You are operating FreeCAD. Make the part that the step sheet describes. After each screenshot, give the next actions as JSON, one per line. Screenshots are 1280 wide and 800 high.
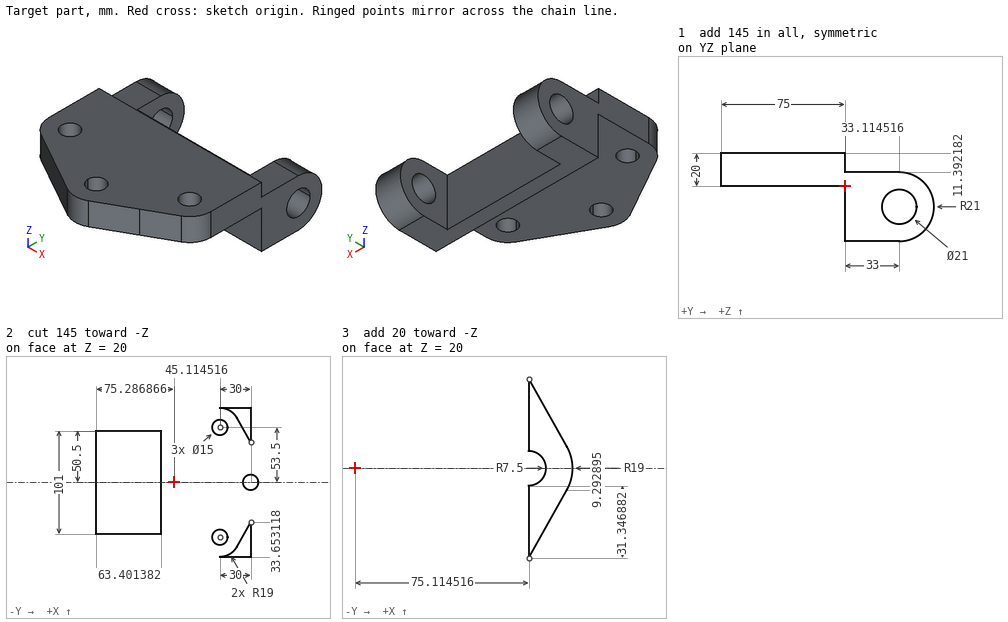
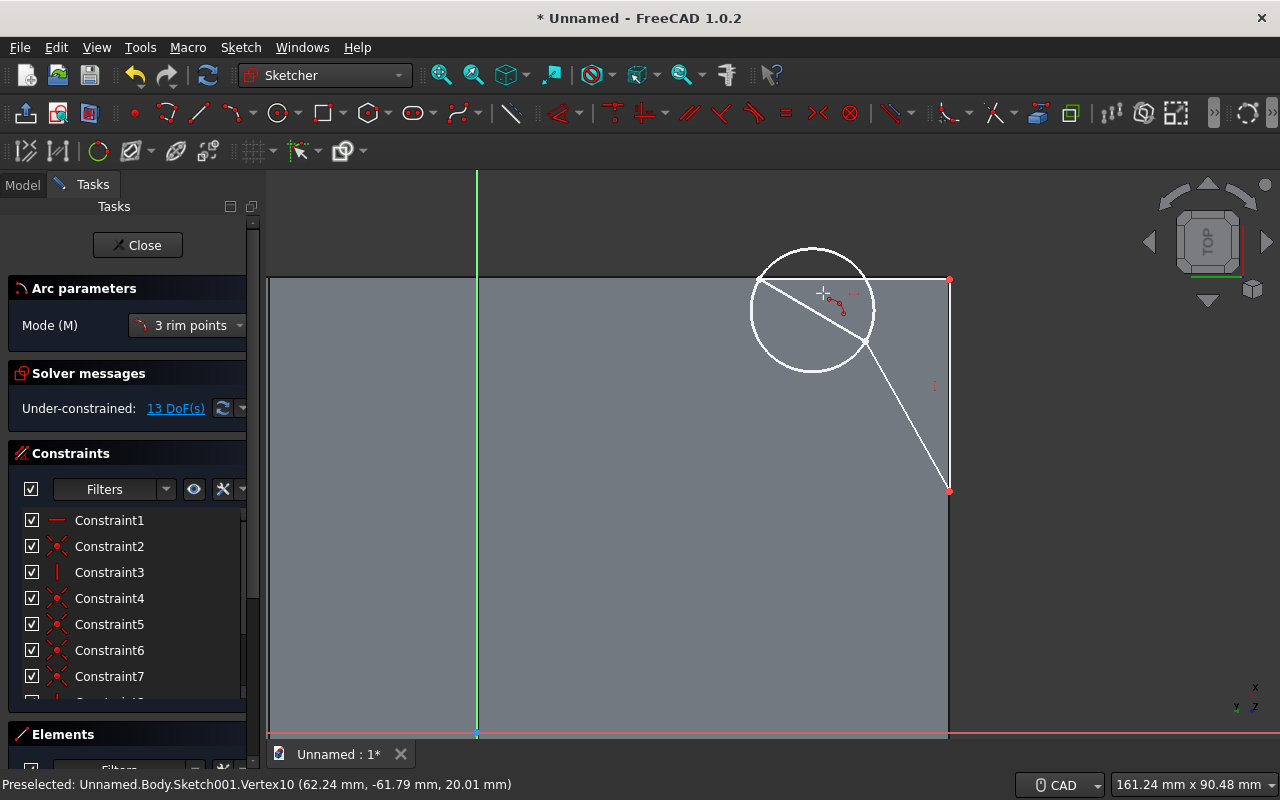
{"action": "left_click", "coordinate": [821, 293]}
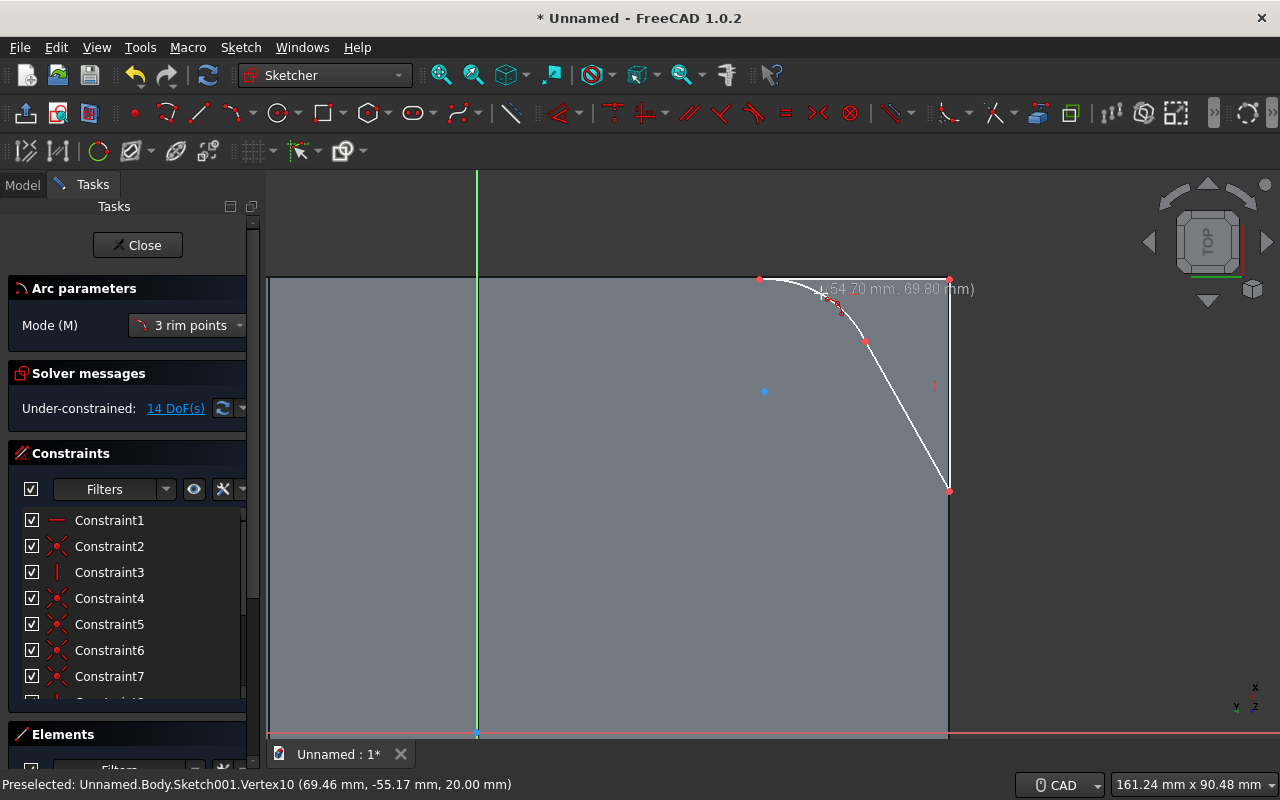
{"action": "left_click", "coordinate": [324, 114]}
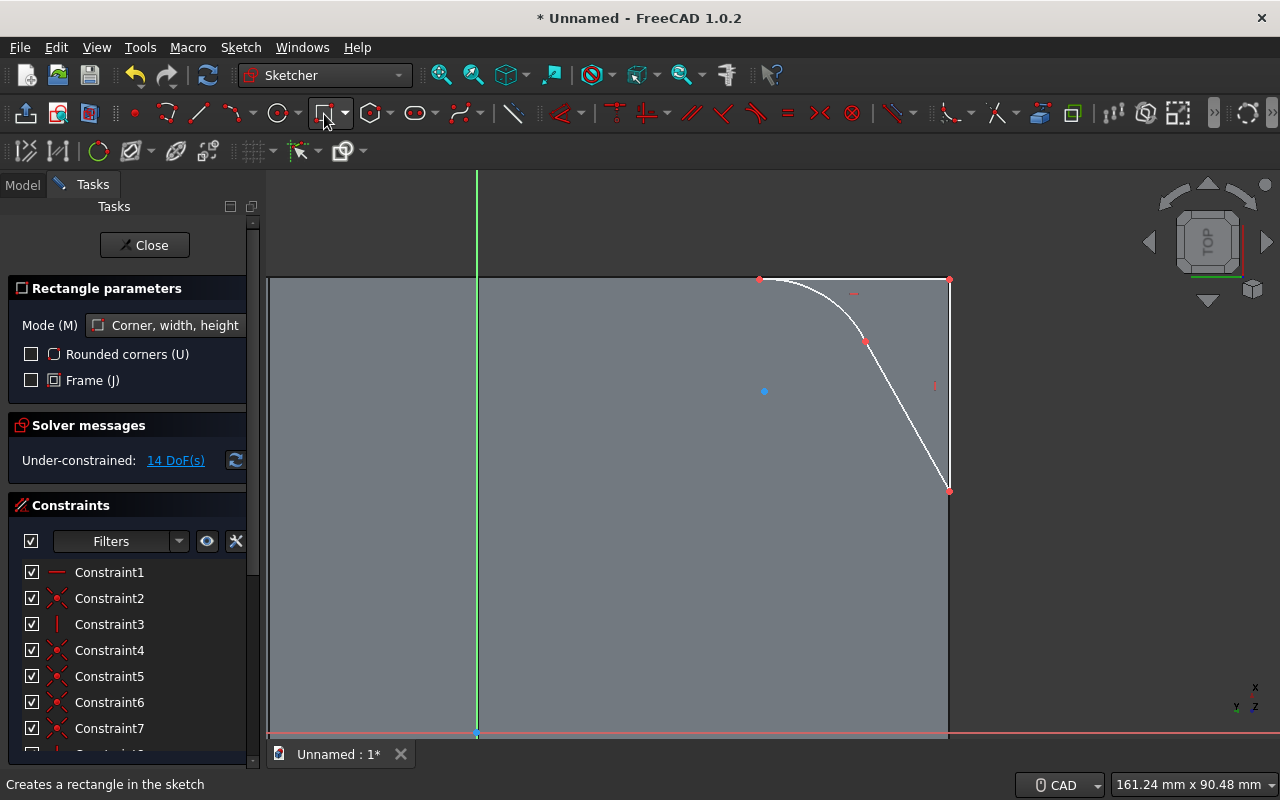
{"action": "scroll", "coordinate": [824, 292], "scroll_direction": "down", "scroll_amount": 5}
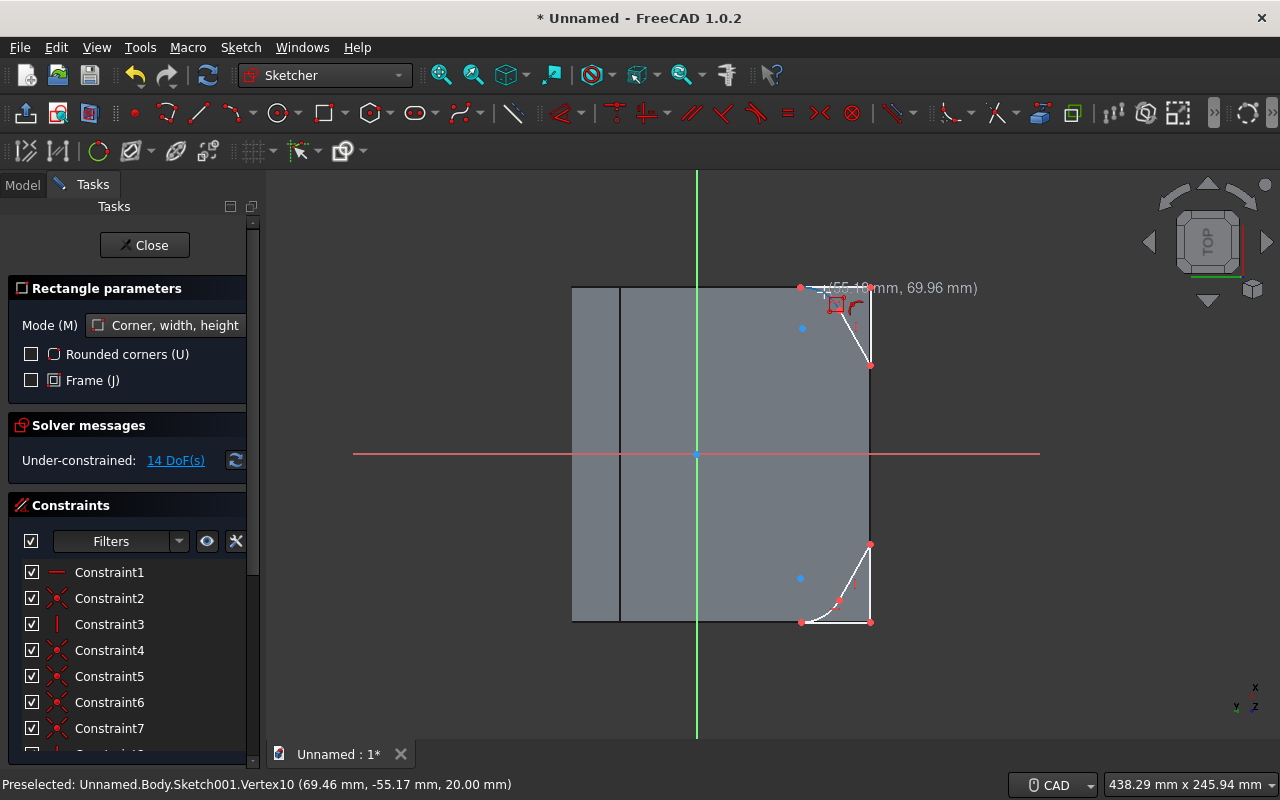
{"action": "left_click", "coordinate": [523, 338]}
{"action": "mouse_move", "coordinate": [669, 571]}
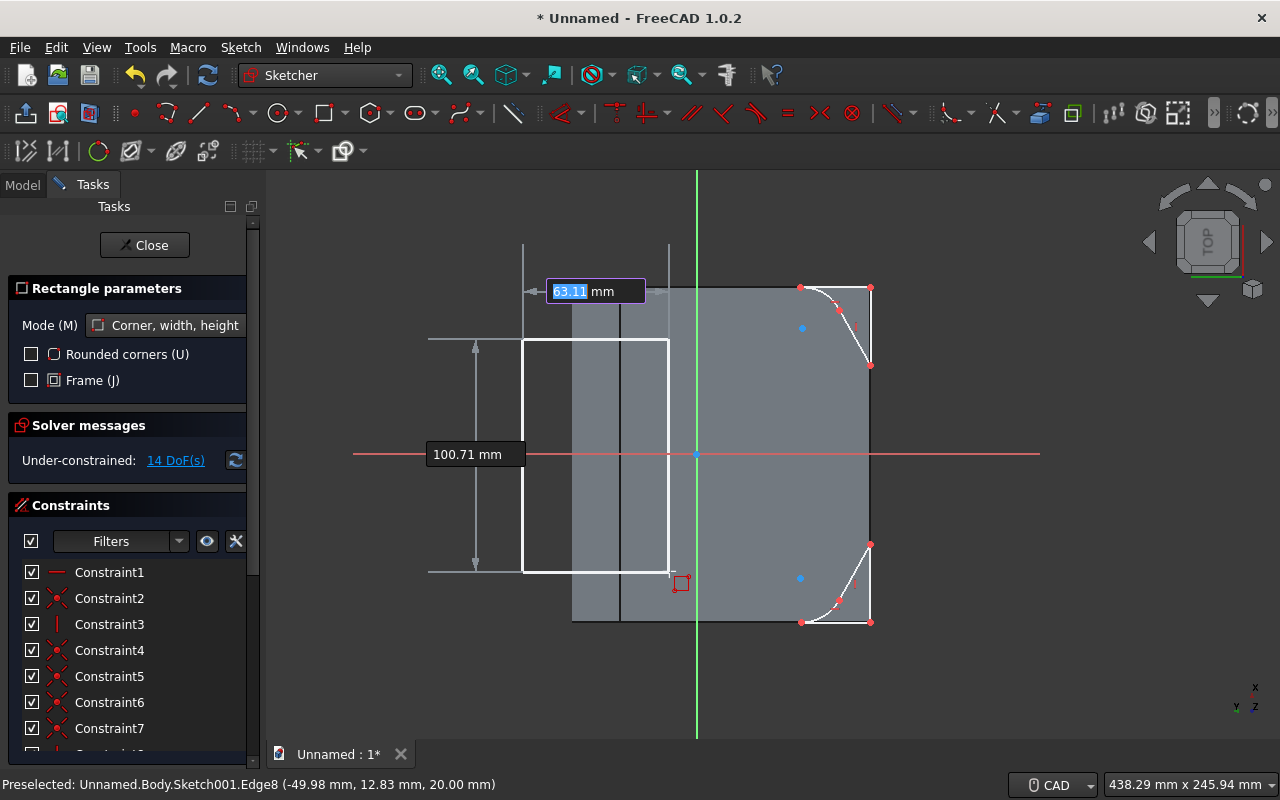
{"action": "type", "text": "63.401382"}
{"action": "key", "text": "Tab"}
{"action": "type", "text": "101"}
{"action": "key", "text": "Return"}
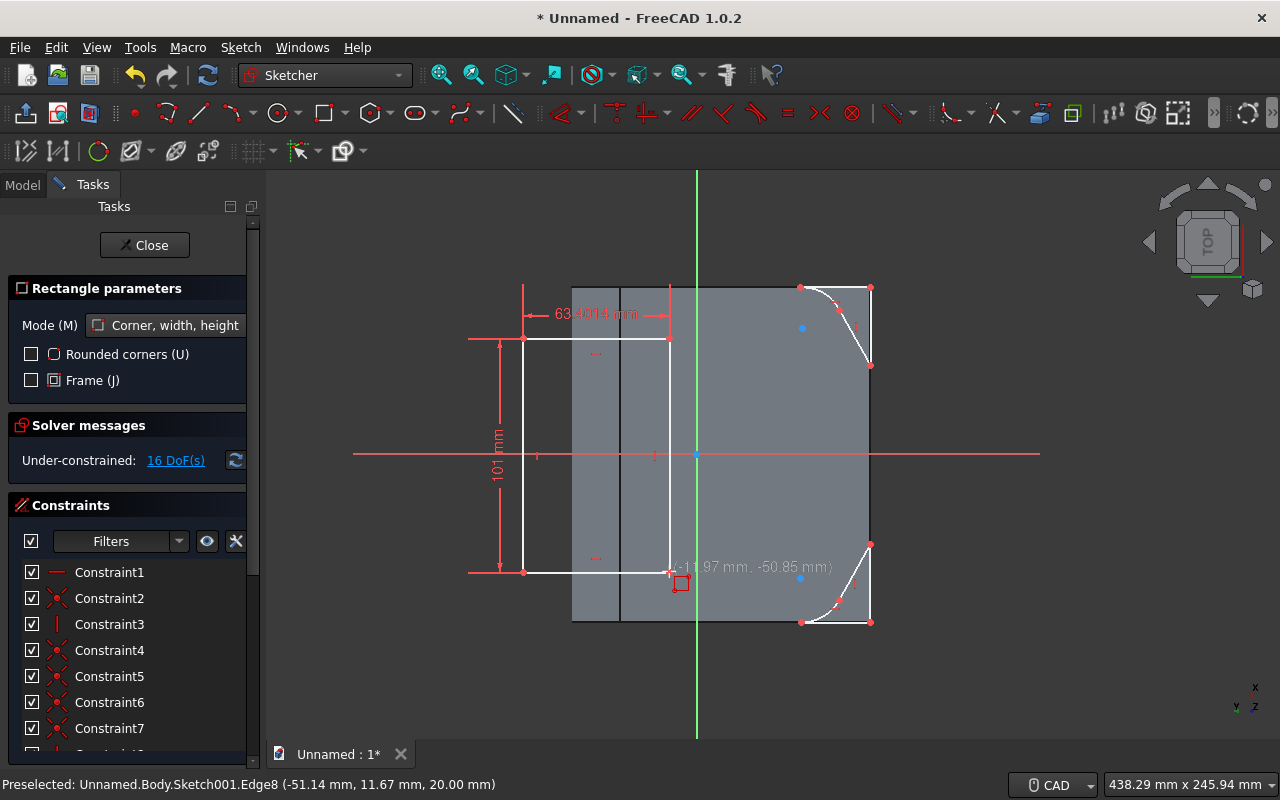
{"action": "left_click", "coordinate": [278, 114]}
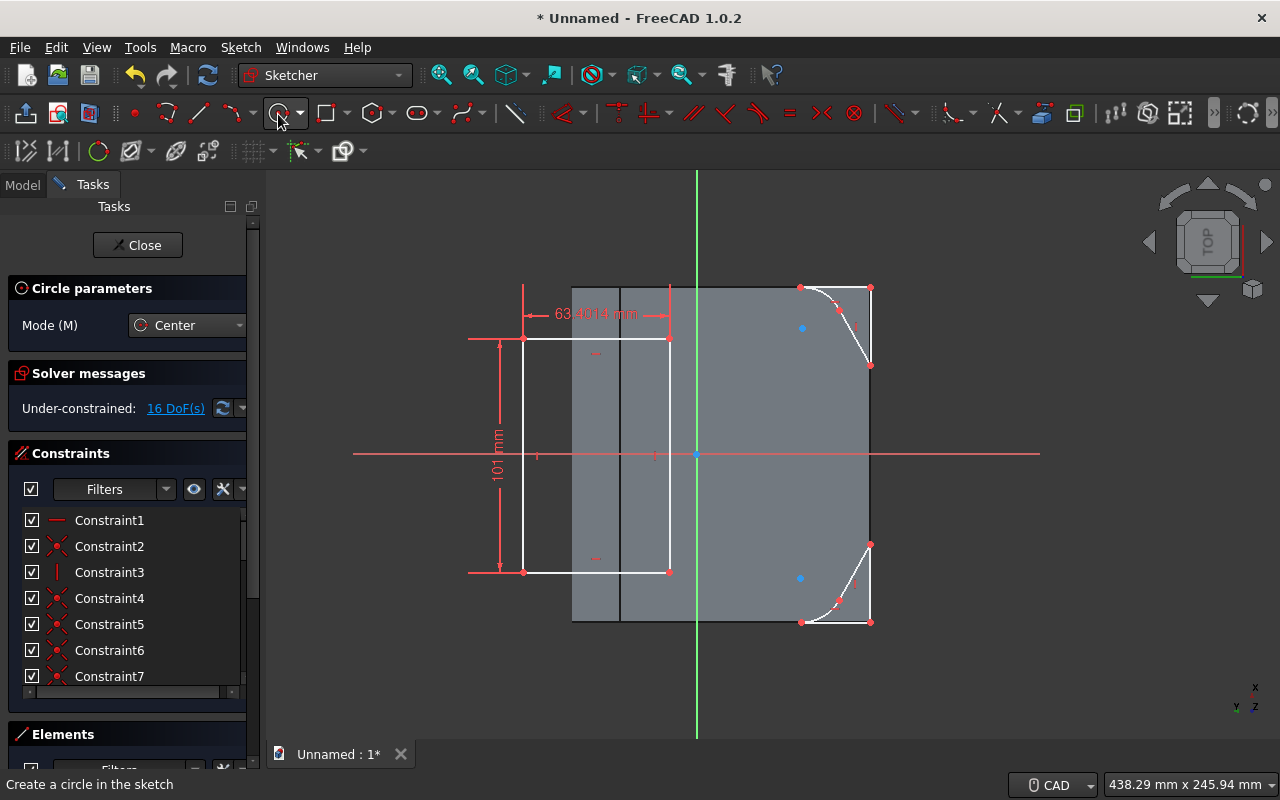
{"action": "scroll", "coordinate": [801, 331], "scroll_direction": "up", "scroll_amount": 2}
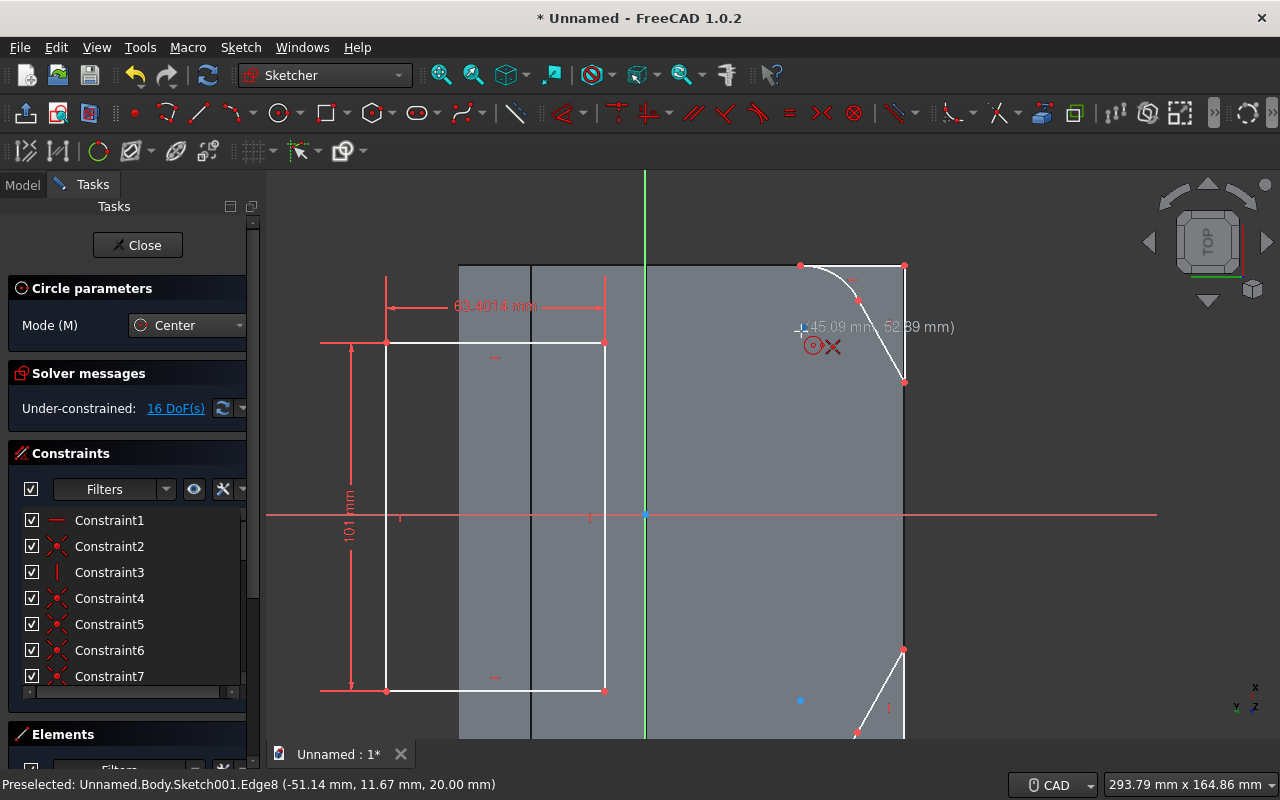
{"action": "left_click", "coordinate": [801, 330]}
{"action": "mouse_move", "coordinate": [819, 312]}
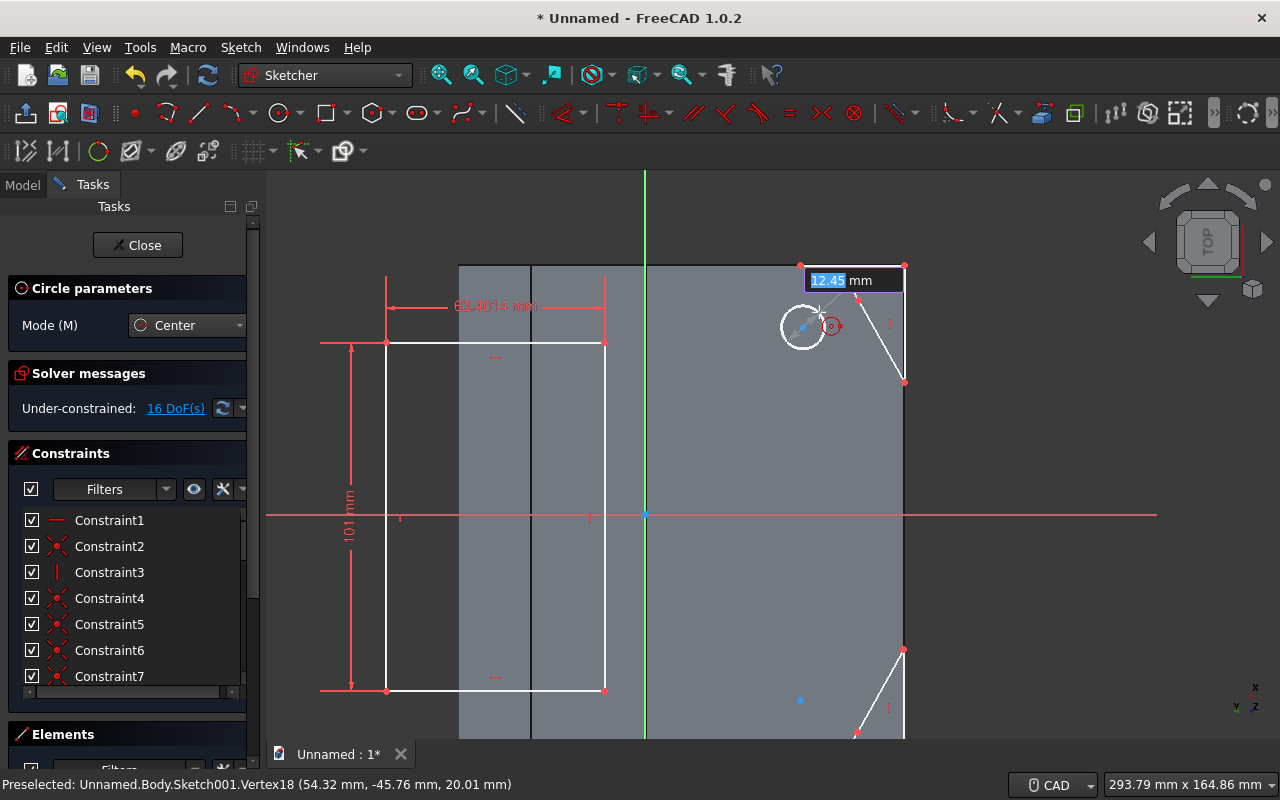
{"action": "type", "text": "15"}
{"action": "key", "text": "Return"}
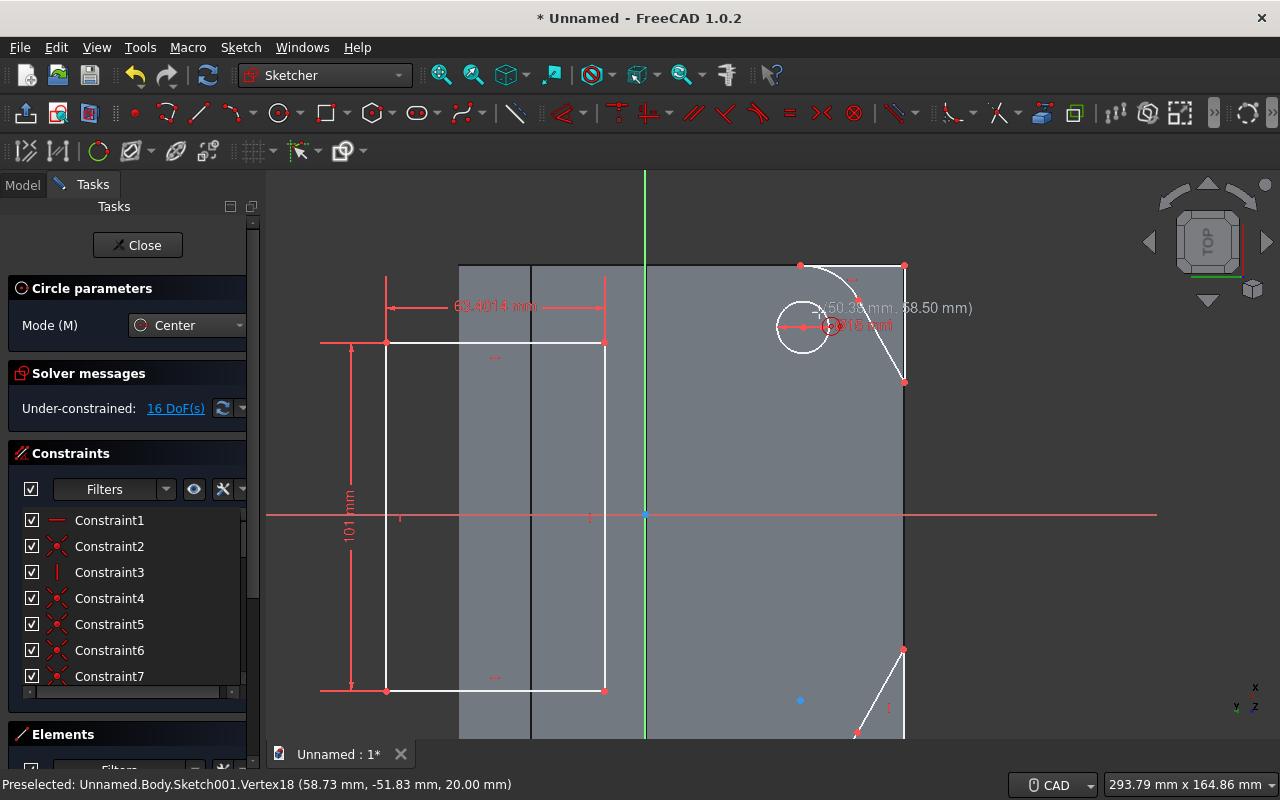
{"action": "left_click", "coordinate": [904, 515]}
{"action": "mouse_move", "coordinate": [923, 497]}